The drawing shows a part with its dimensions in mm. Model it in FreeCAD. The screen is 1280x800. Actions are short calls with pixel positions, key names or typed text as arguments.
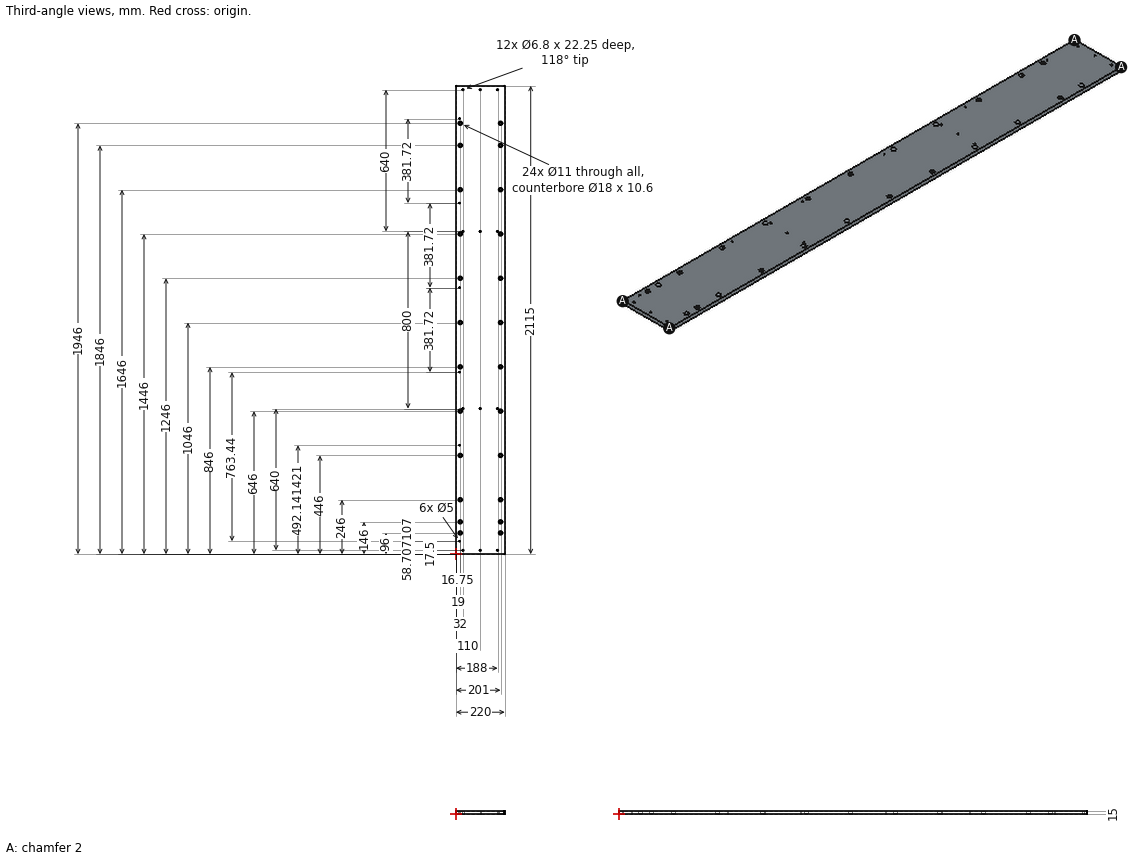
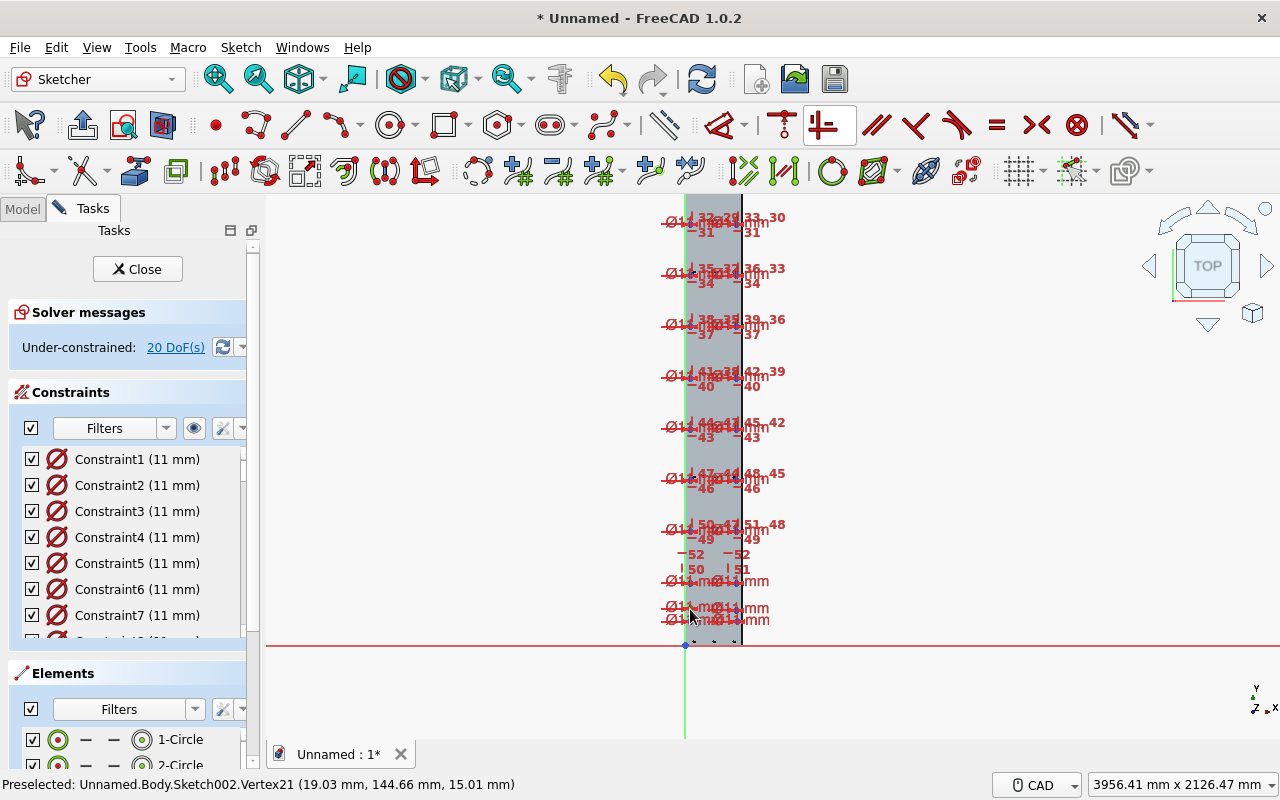
click(850, 126)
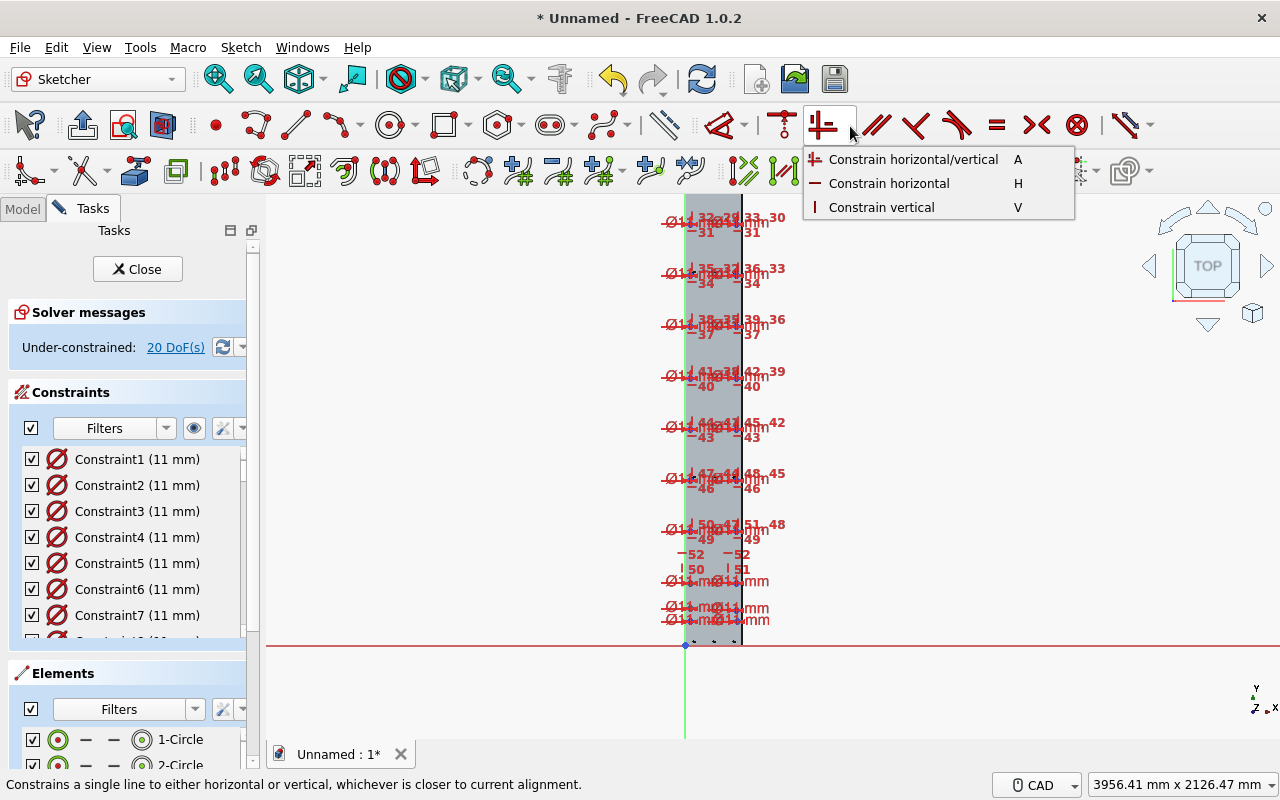
click(939, 207)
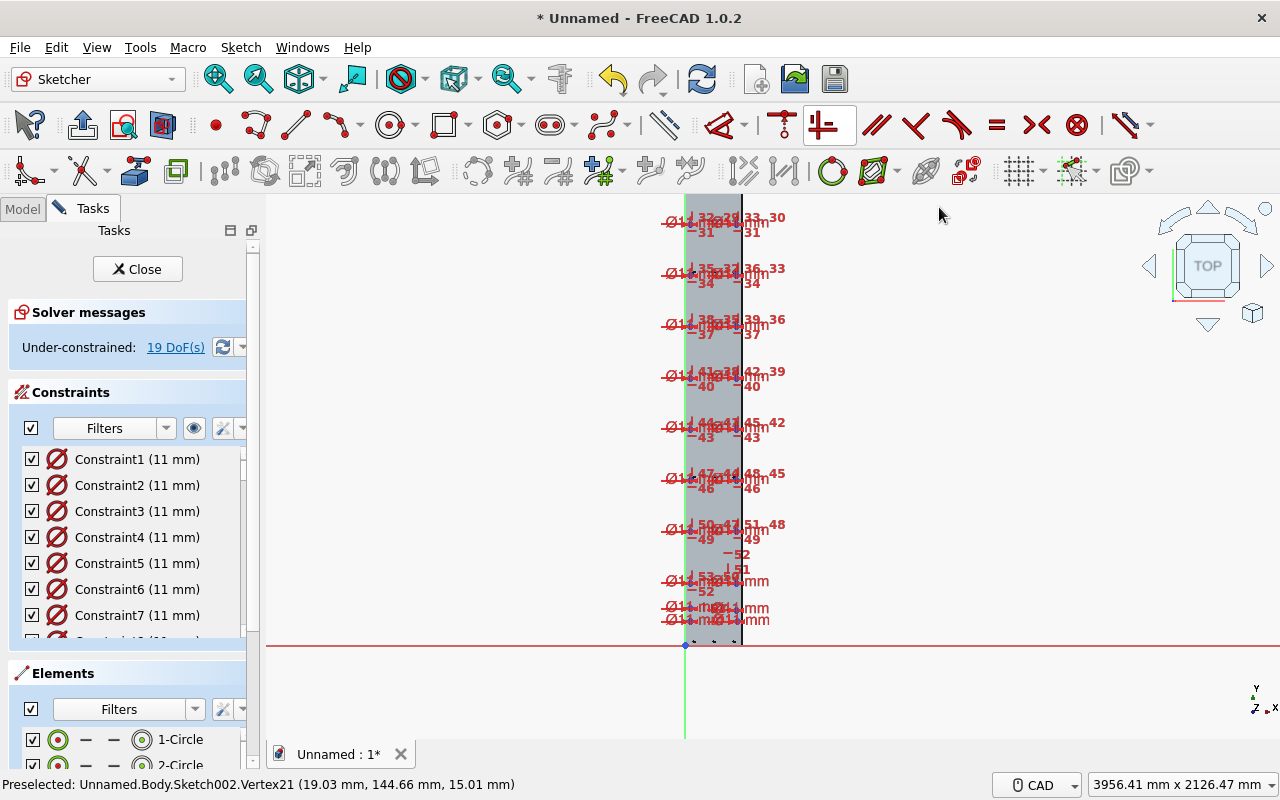
click(736, 583)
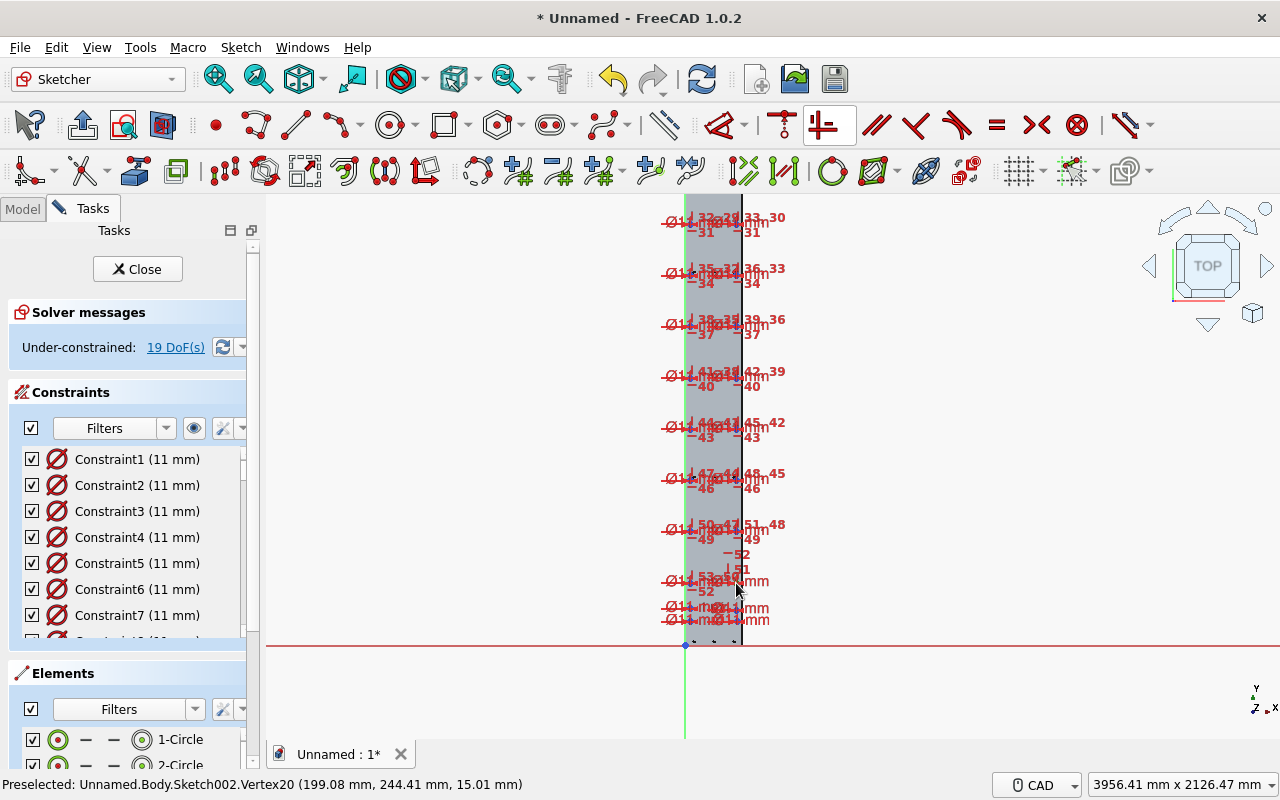
click(736, 610)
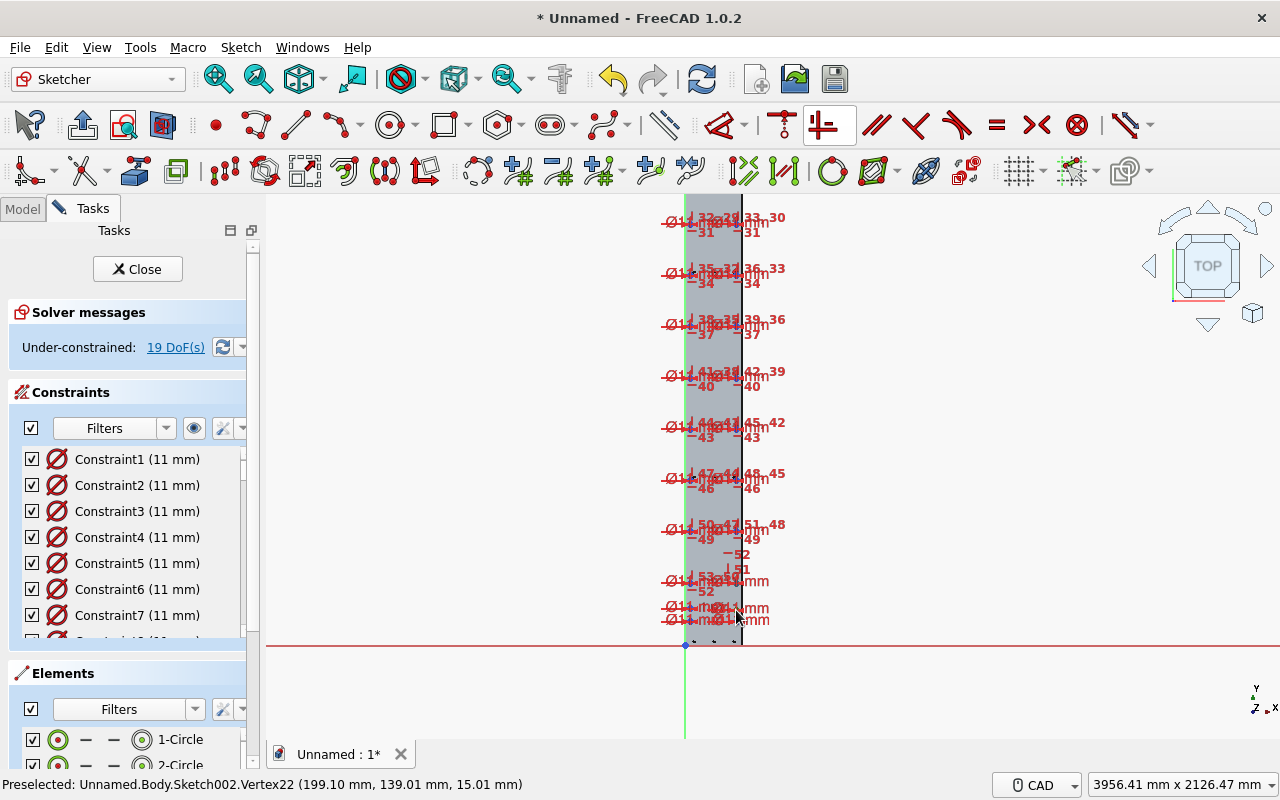
click(850, 126)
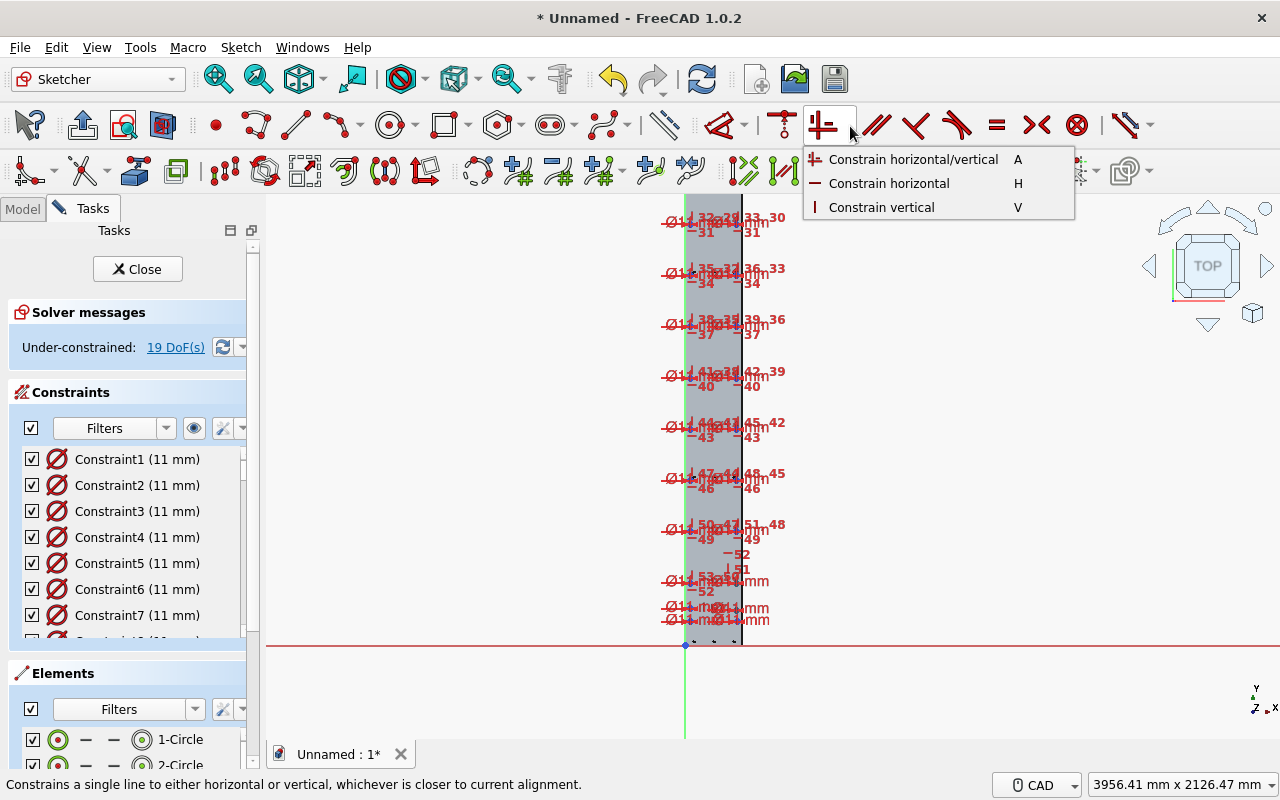
click(939, 207)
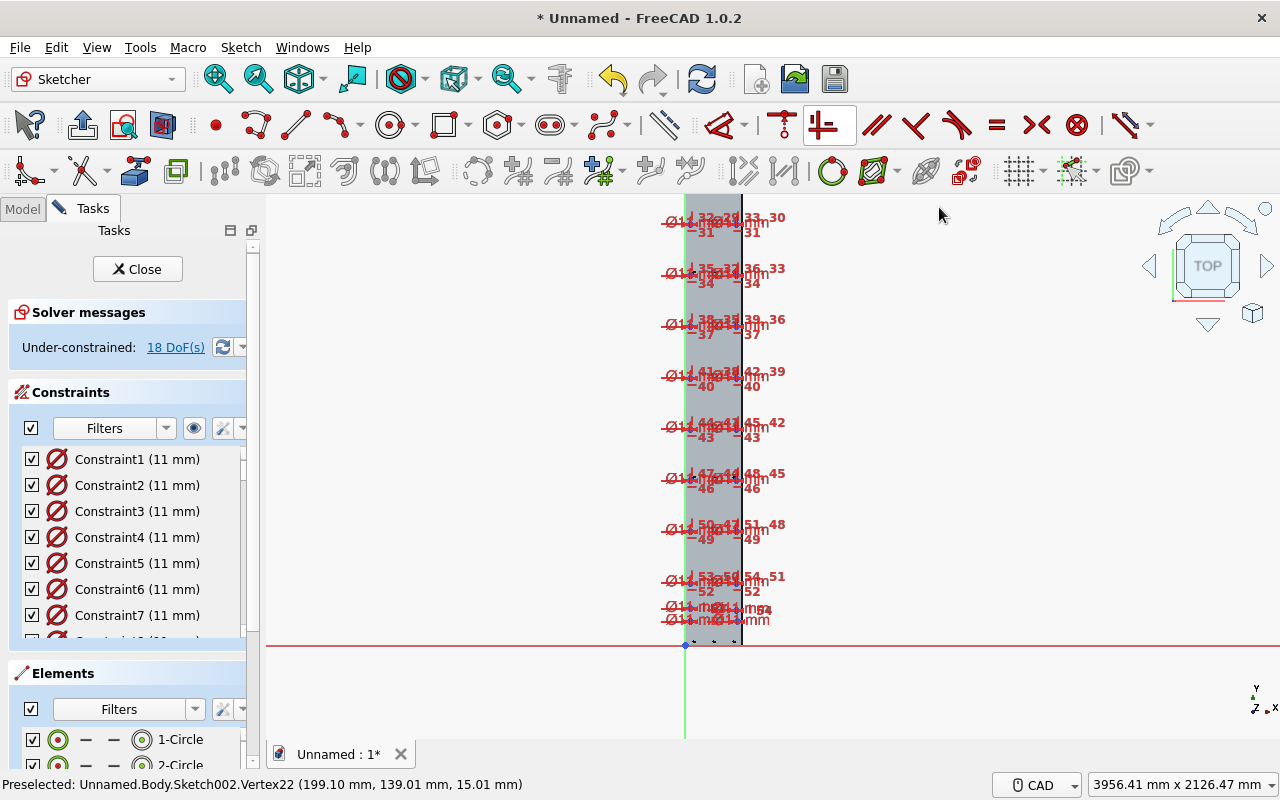
click(690, 609)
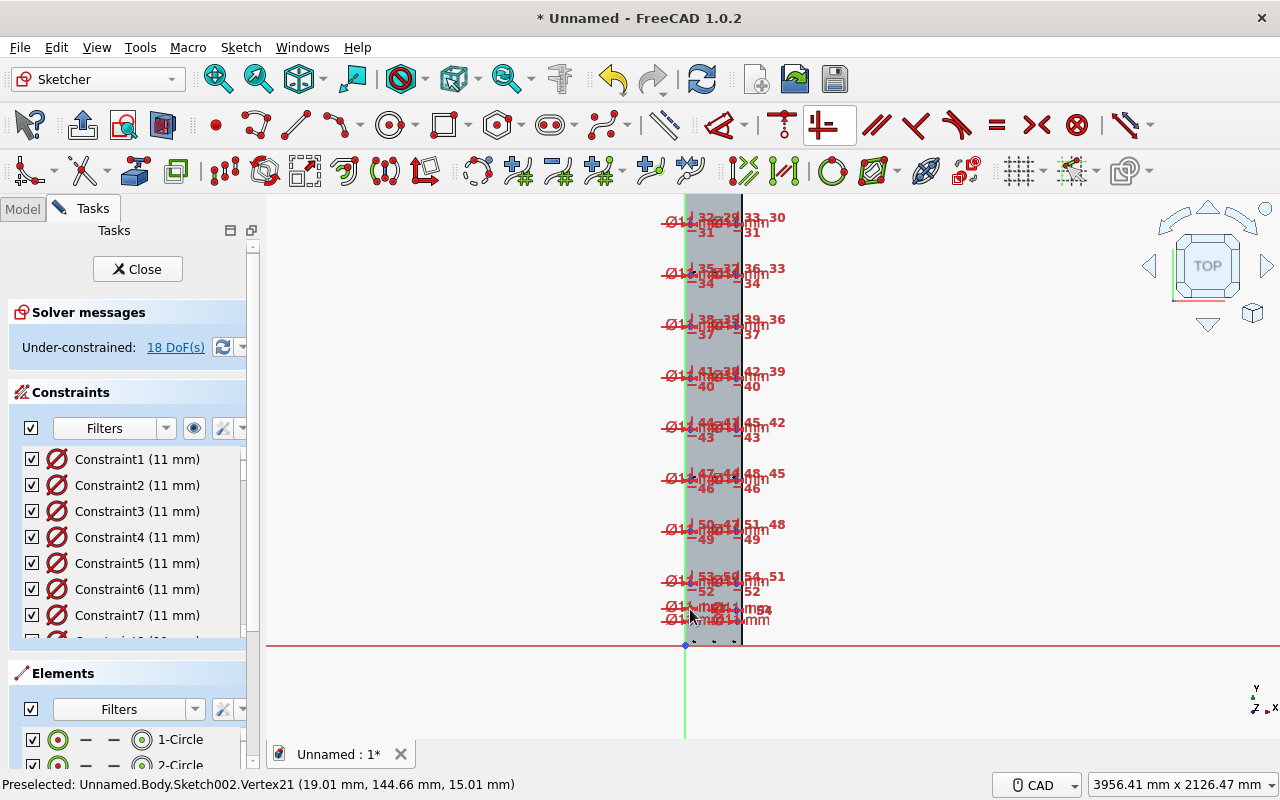
click(736, 610)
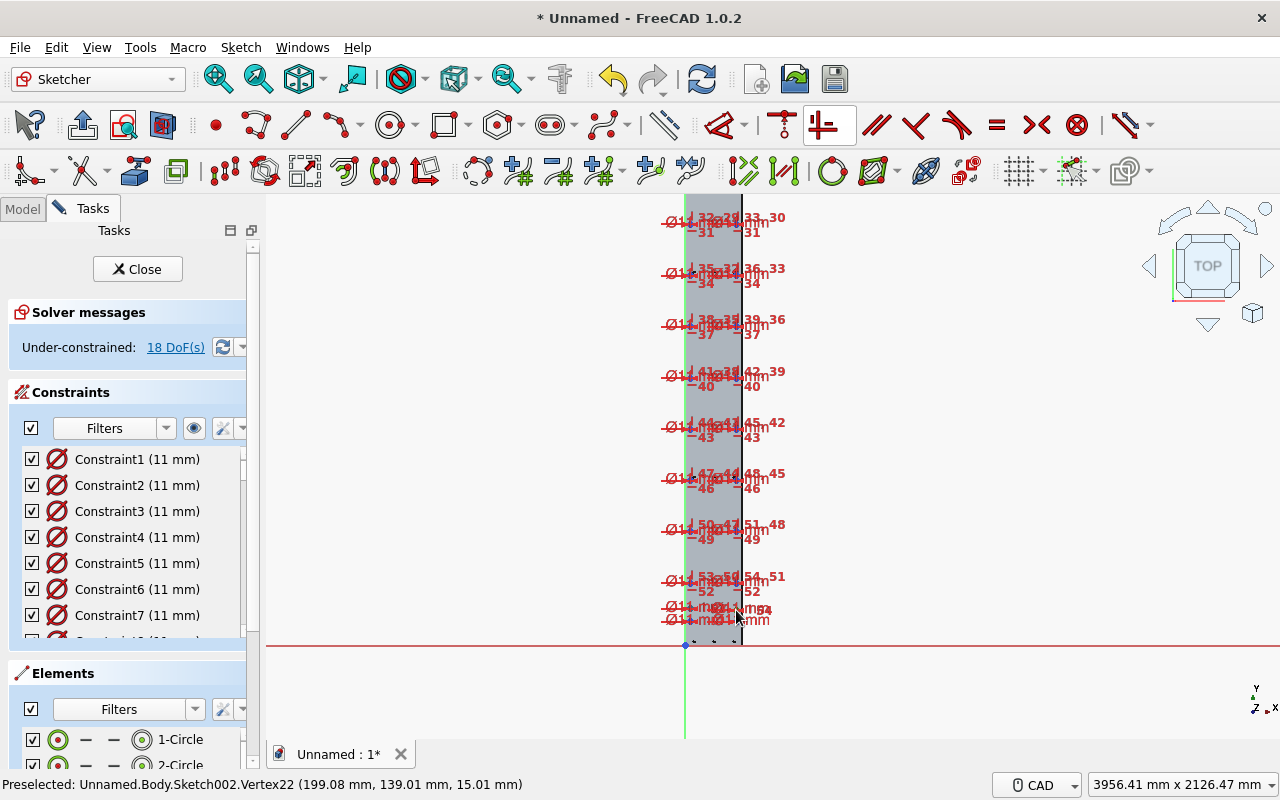
click(850, 126)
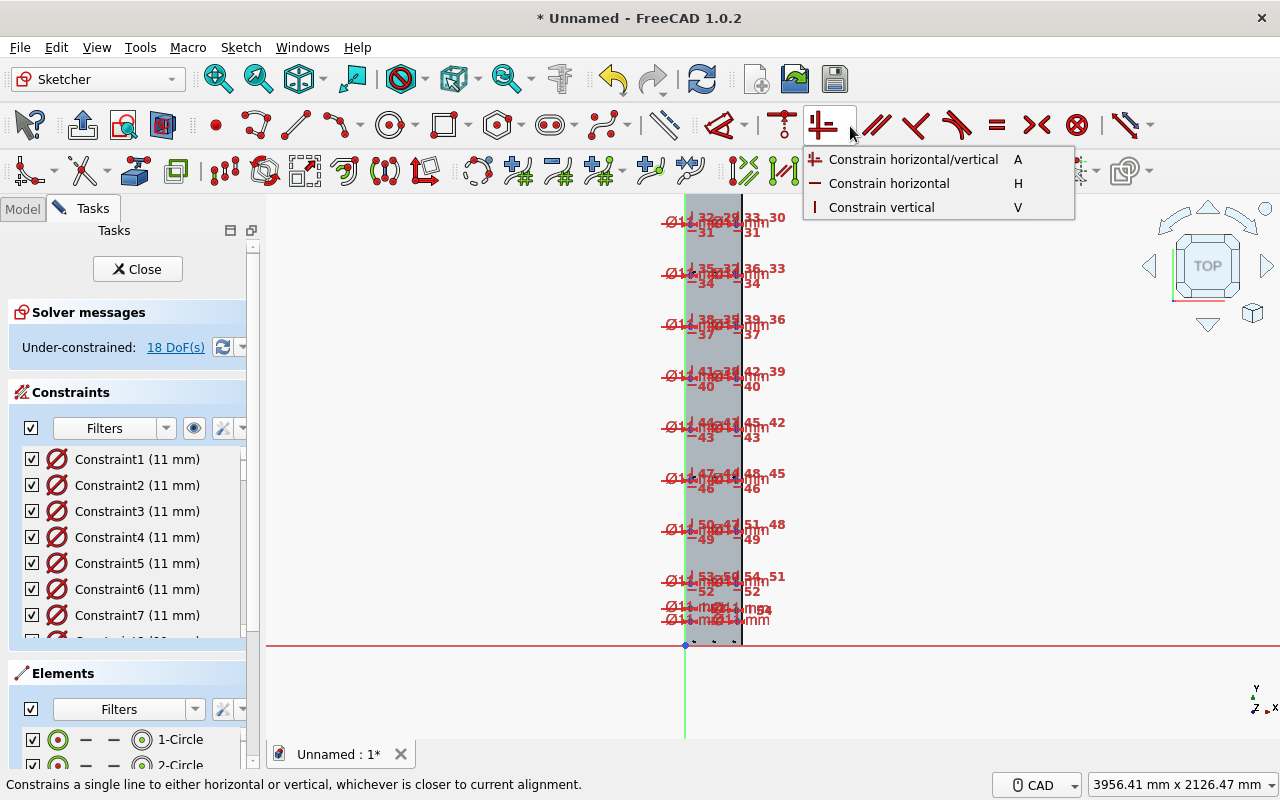
click(939, 183)